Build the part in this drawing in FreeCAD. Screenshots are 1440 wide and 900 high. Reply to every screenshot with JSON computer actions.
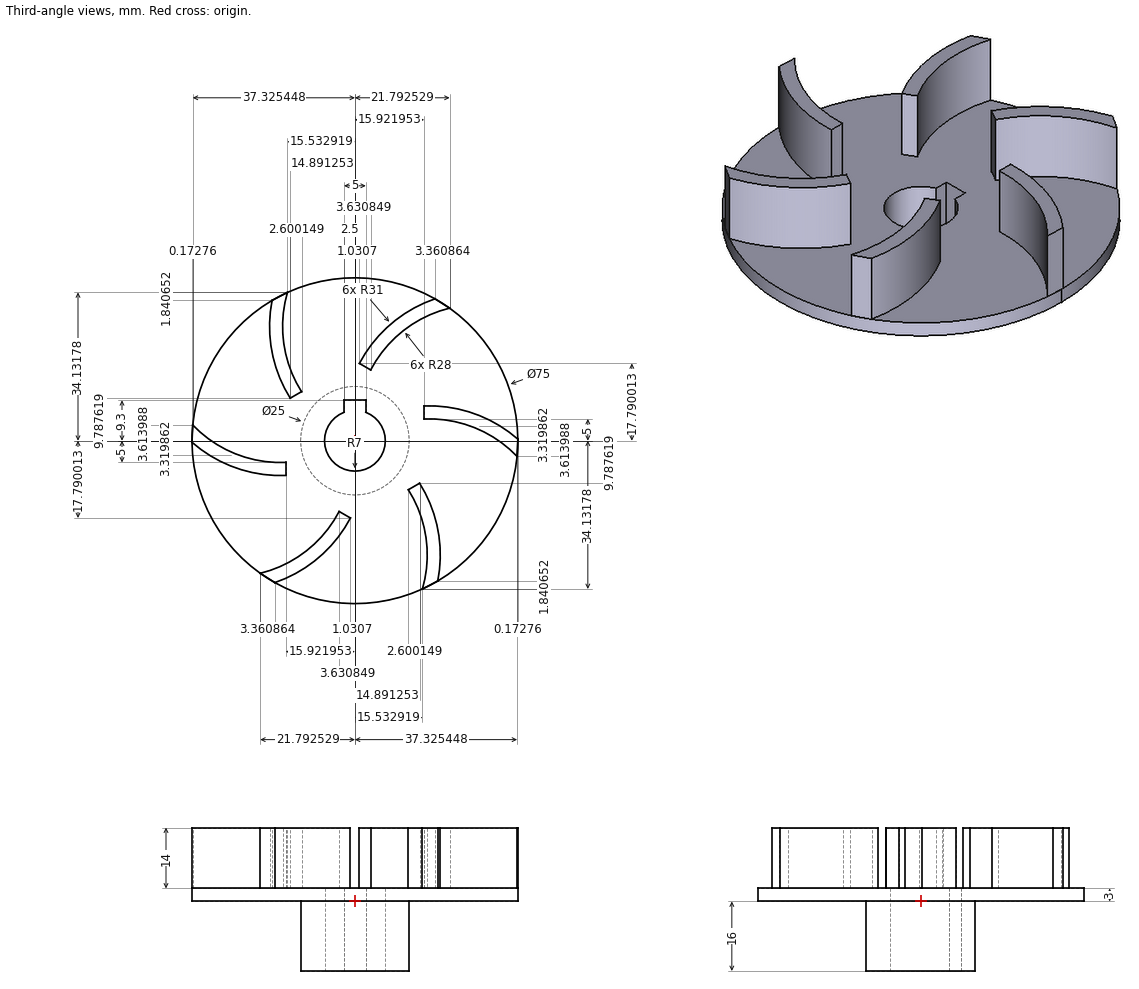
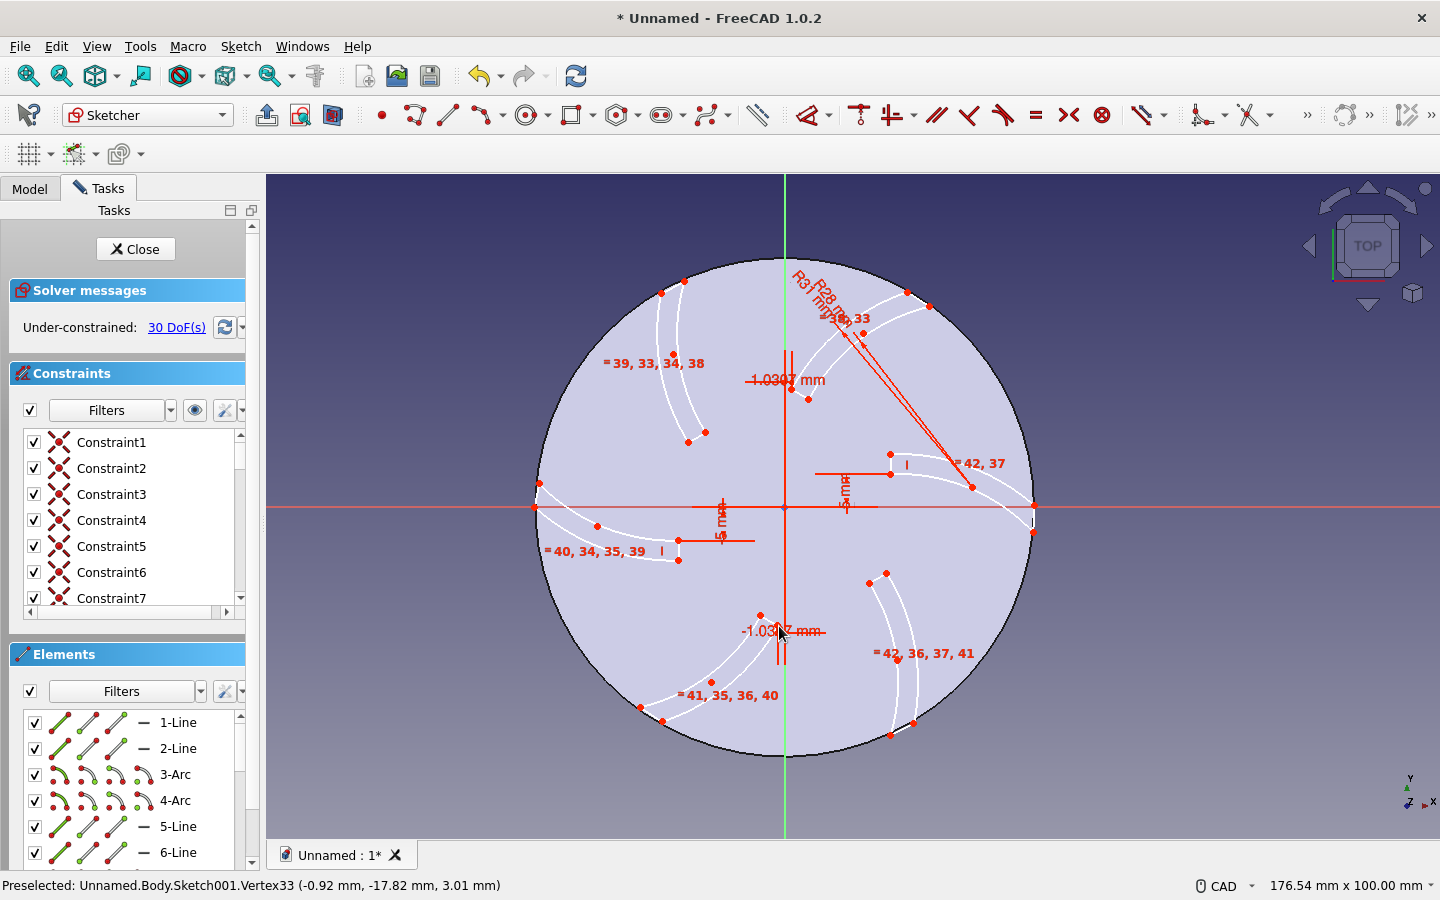
{"action": "scroll", "coordinate": [538, 491], "scroll_direction": "up", "scroll_amount": 18}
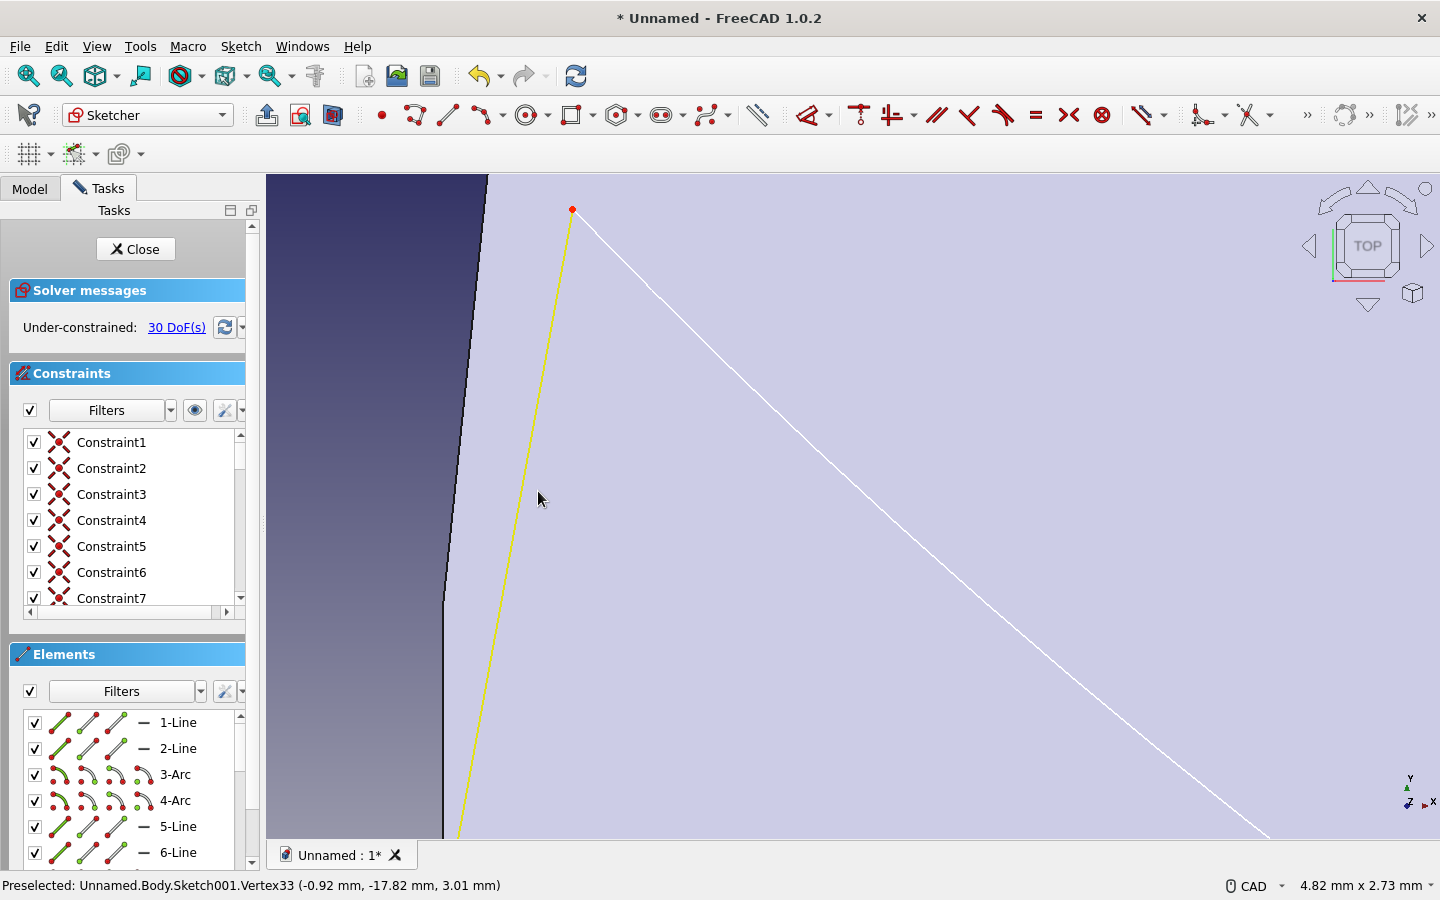
{"action": "left_click", "coordinate": [526, 468]}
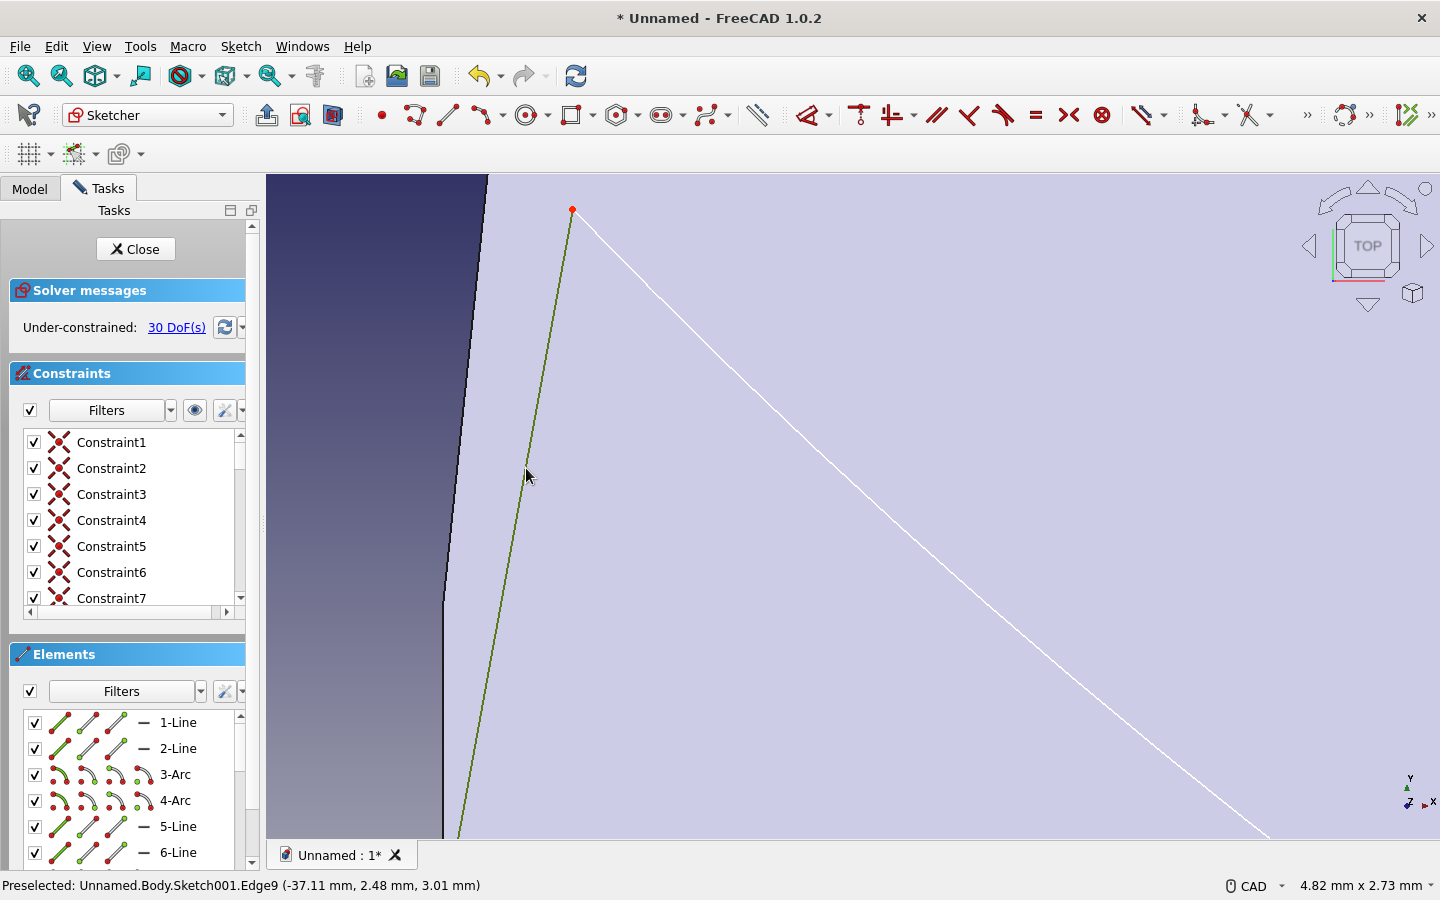
{"action": "key", "text": "l"}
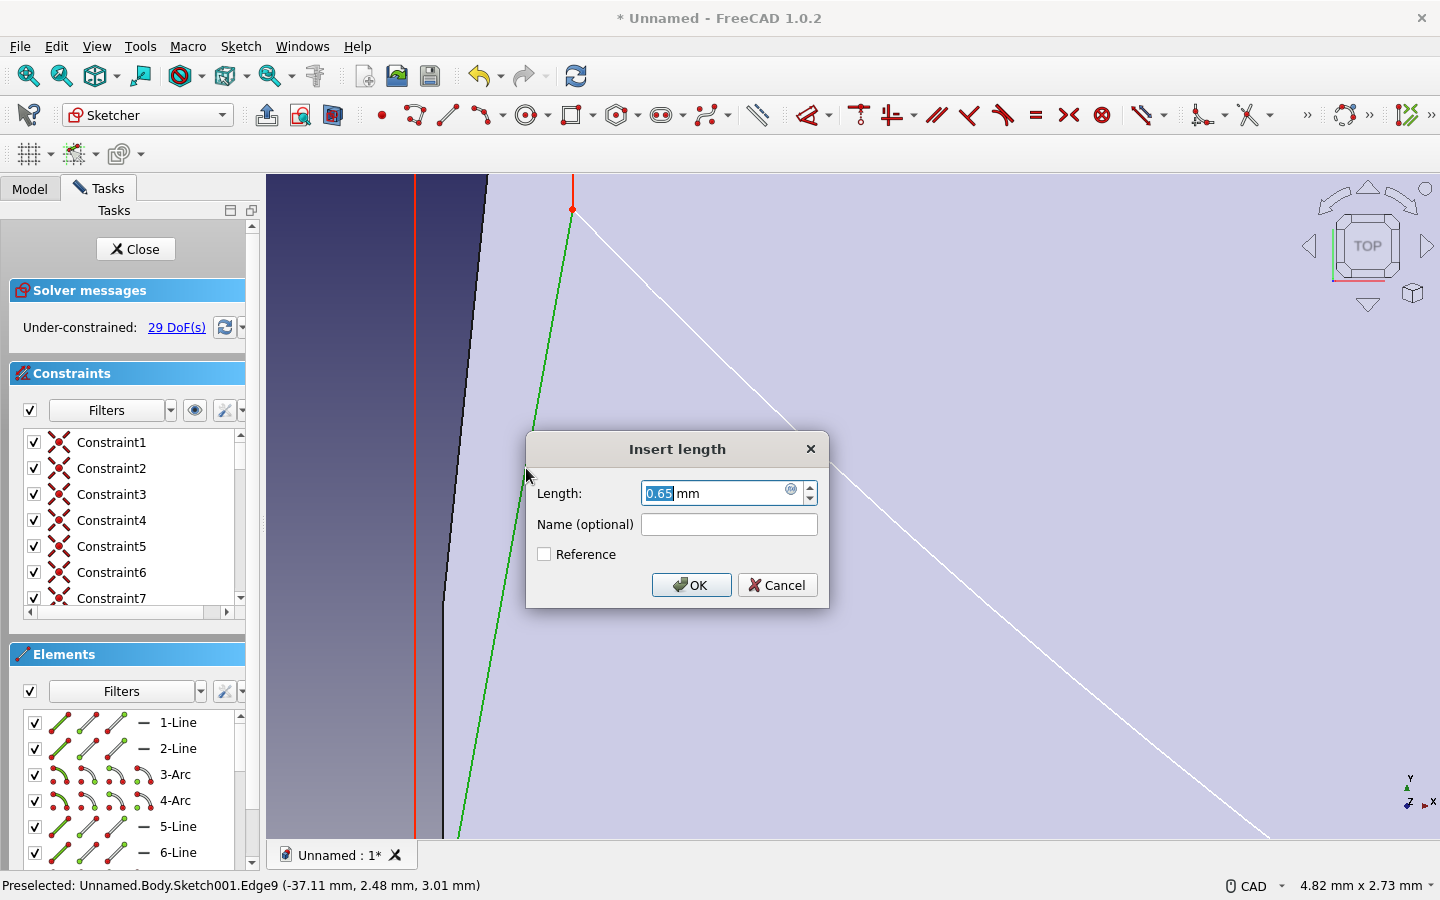
{"action": "type", "text": "0.17276"}
{"action": "key", "text": "Return"}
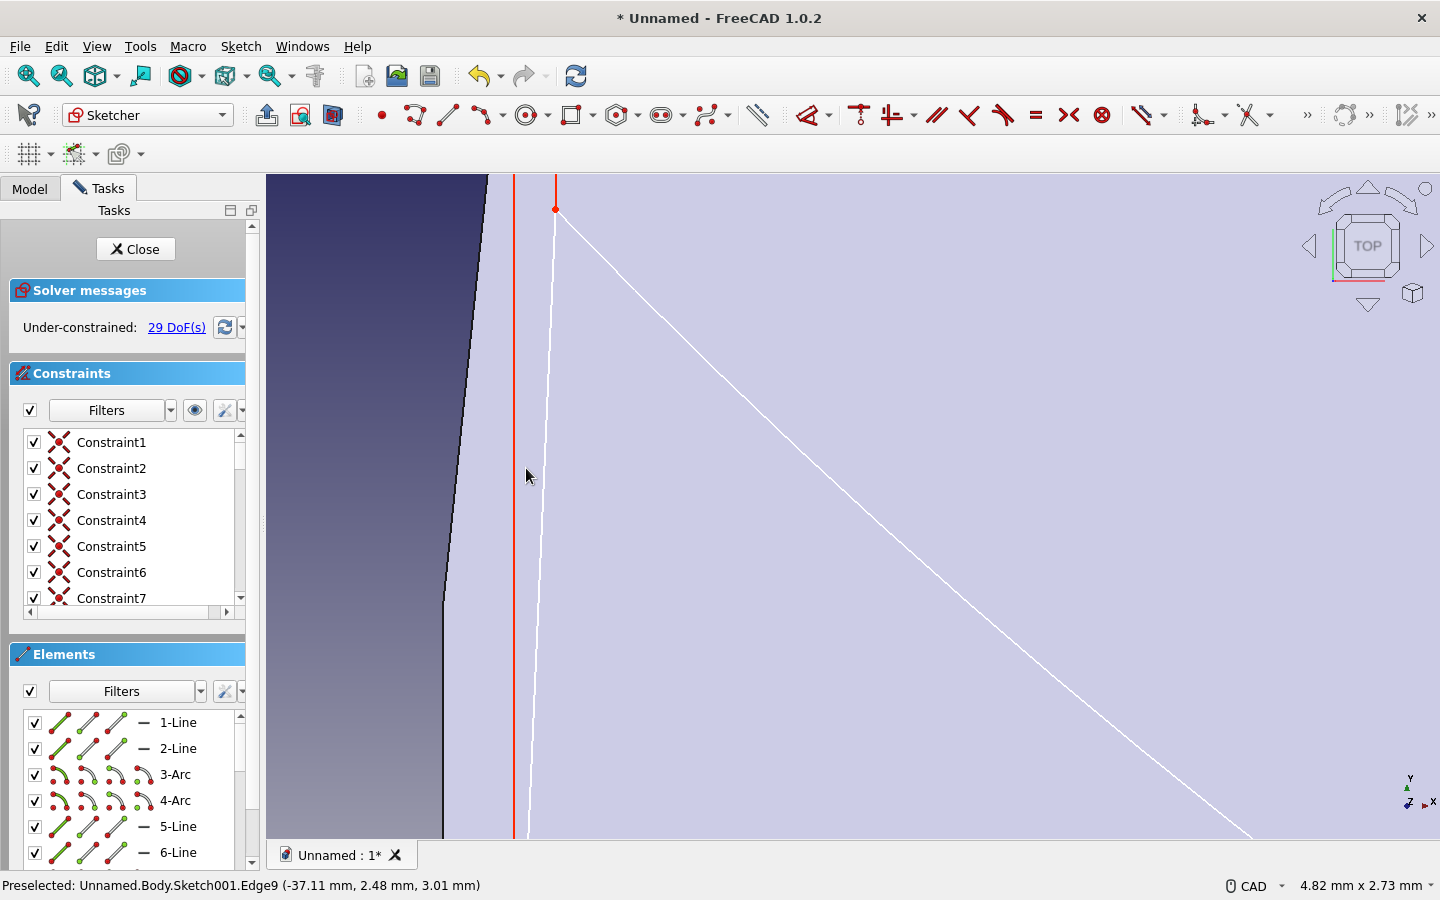
{"action": "scroll", "coordinate": [482, 487], "scroll_direction": "down", "scroll_amount": 17}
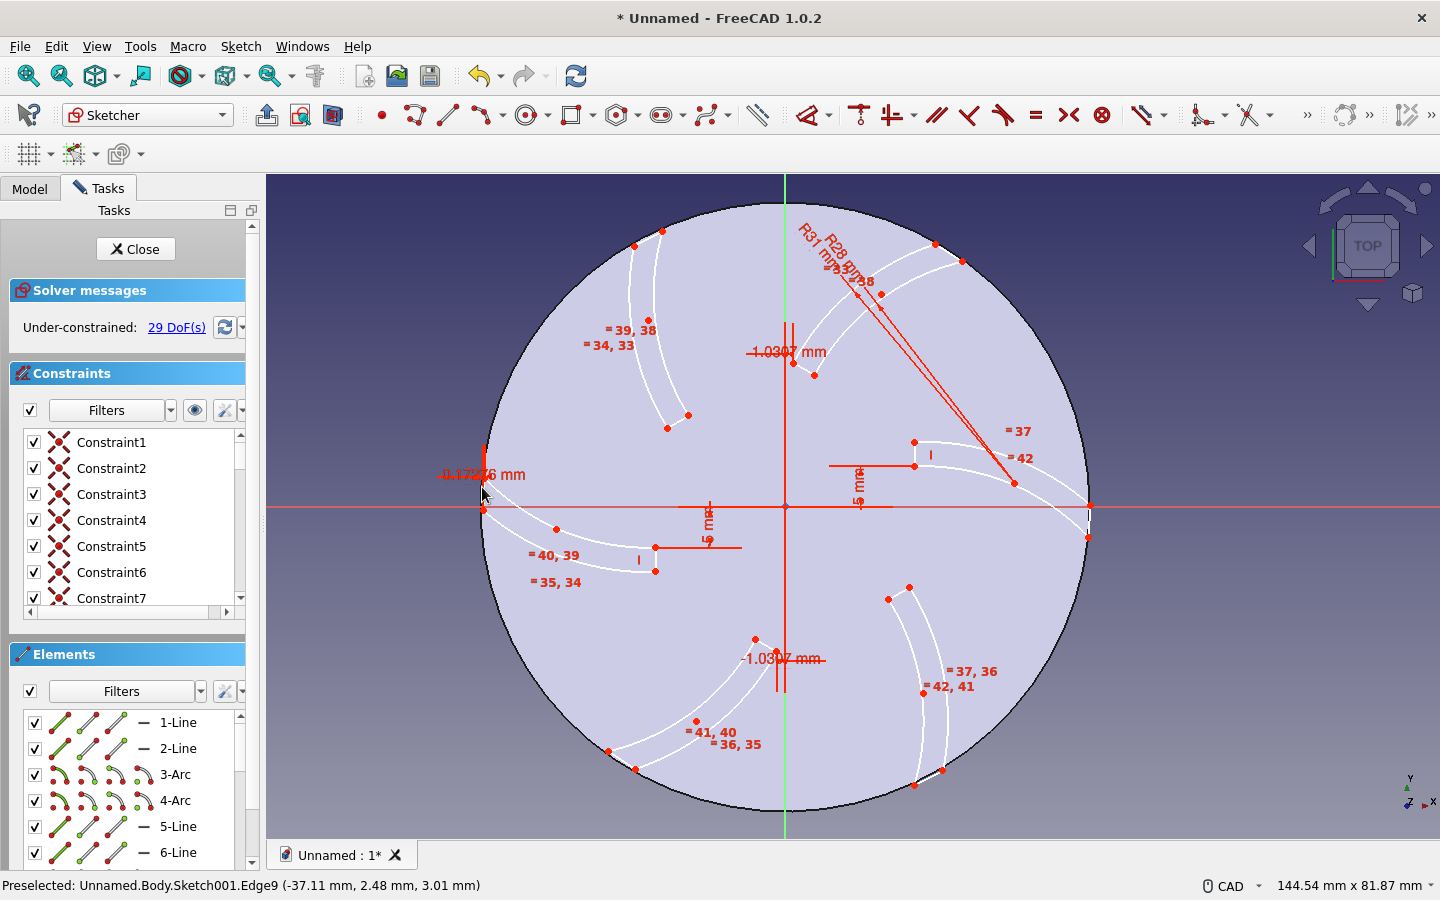
{"action": "scroll", "coordinate": [1089, 528], "scroll_direction": "up", "scroll_amount": 17}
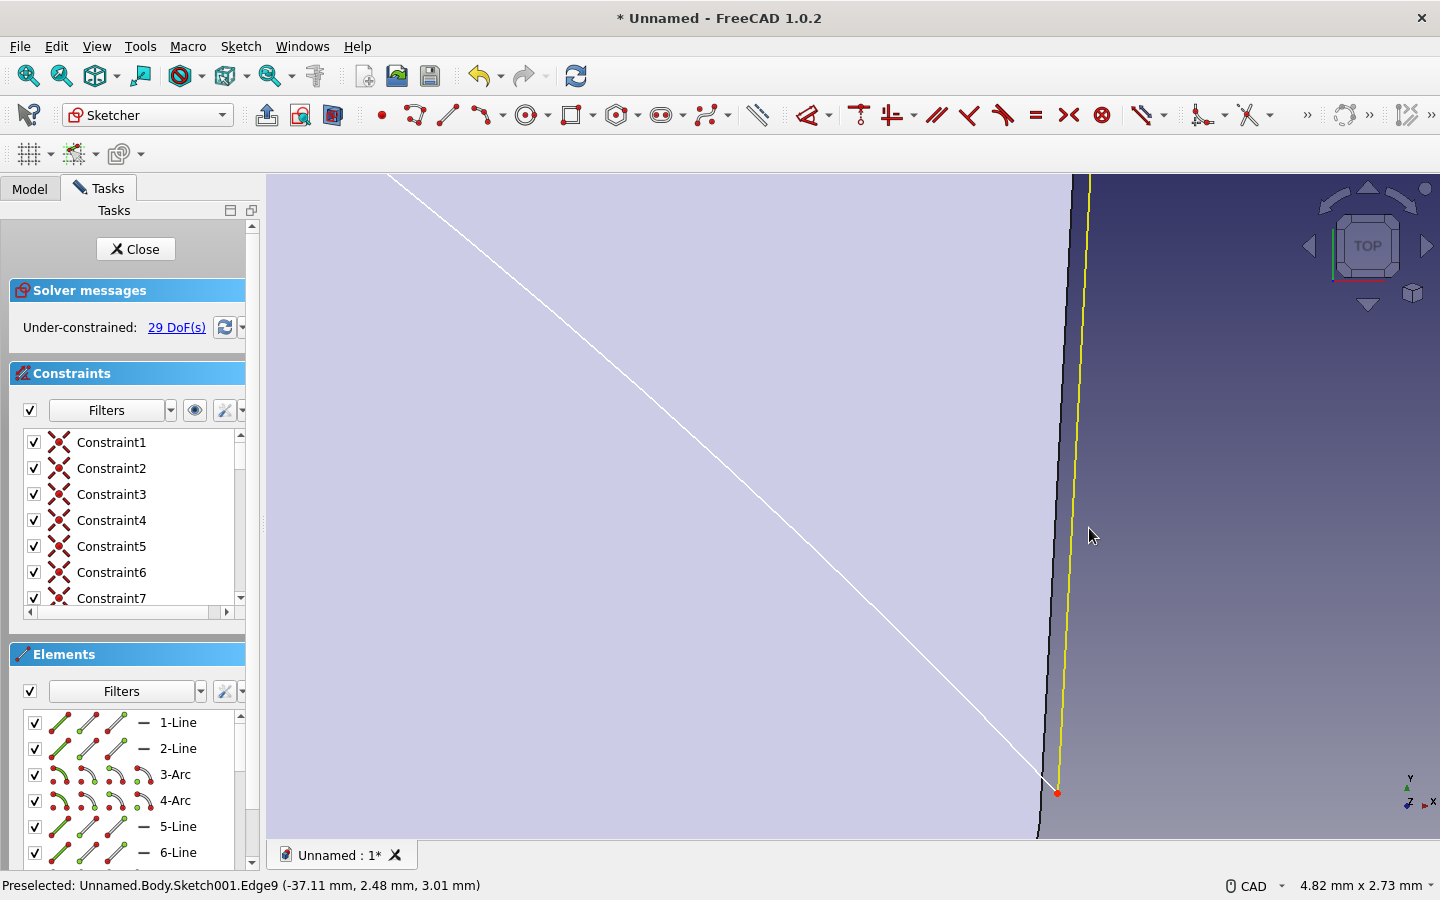
{"action": "left_click", "coordinate": [1073, 504]}